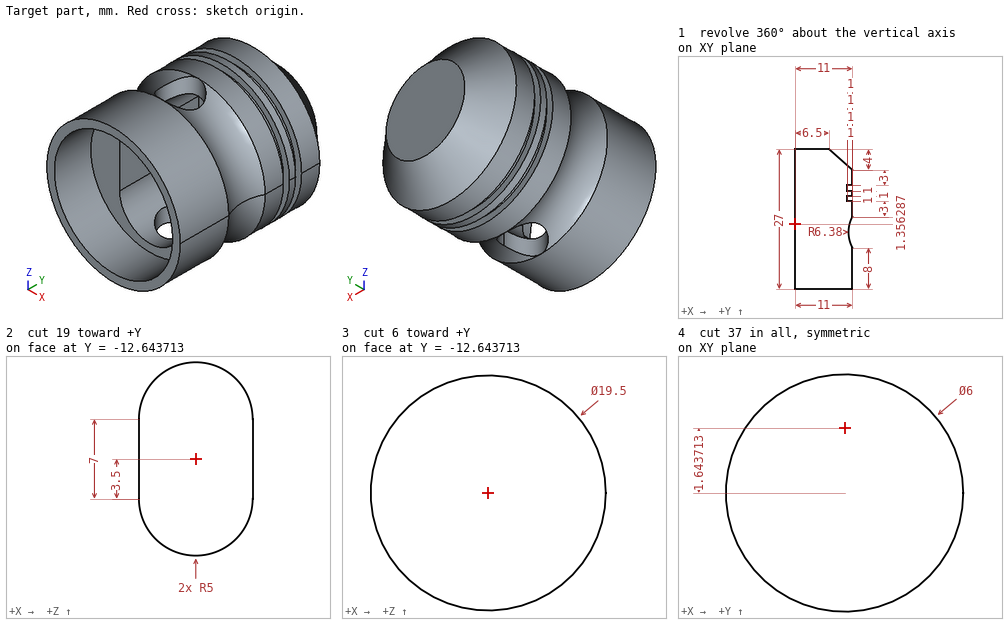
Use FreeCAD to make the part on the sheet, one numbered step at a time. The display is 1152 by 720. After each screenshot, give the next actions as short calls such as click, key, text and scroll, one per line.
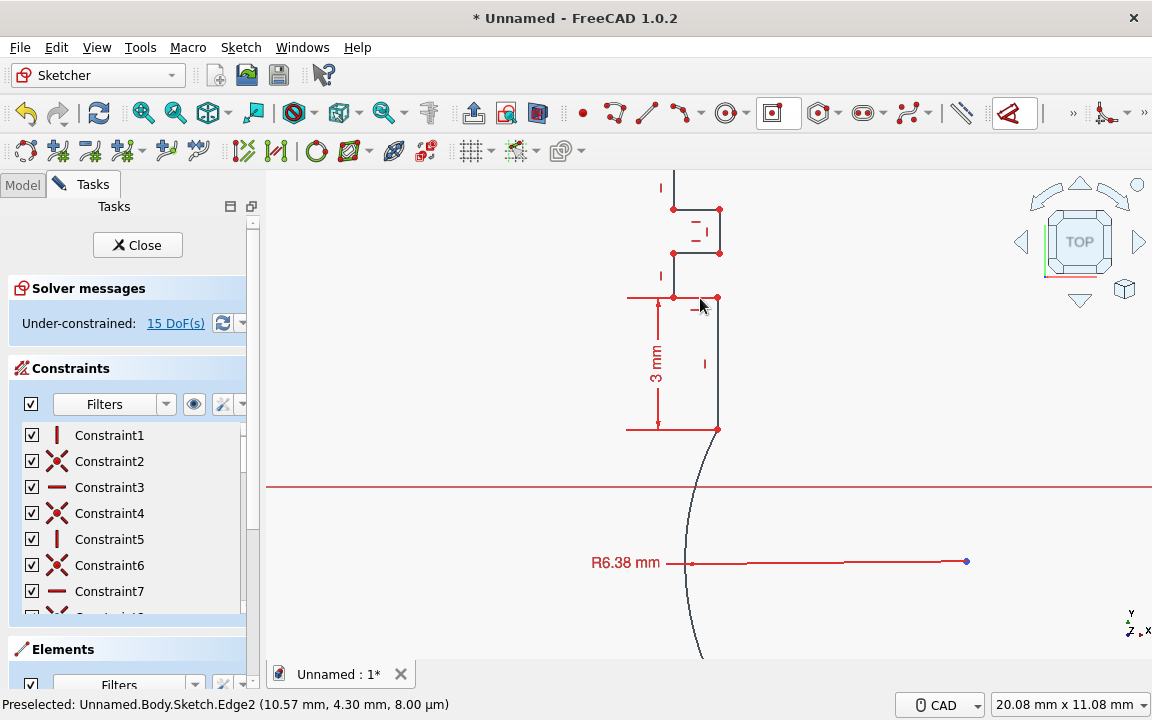
click(1032, 114)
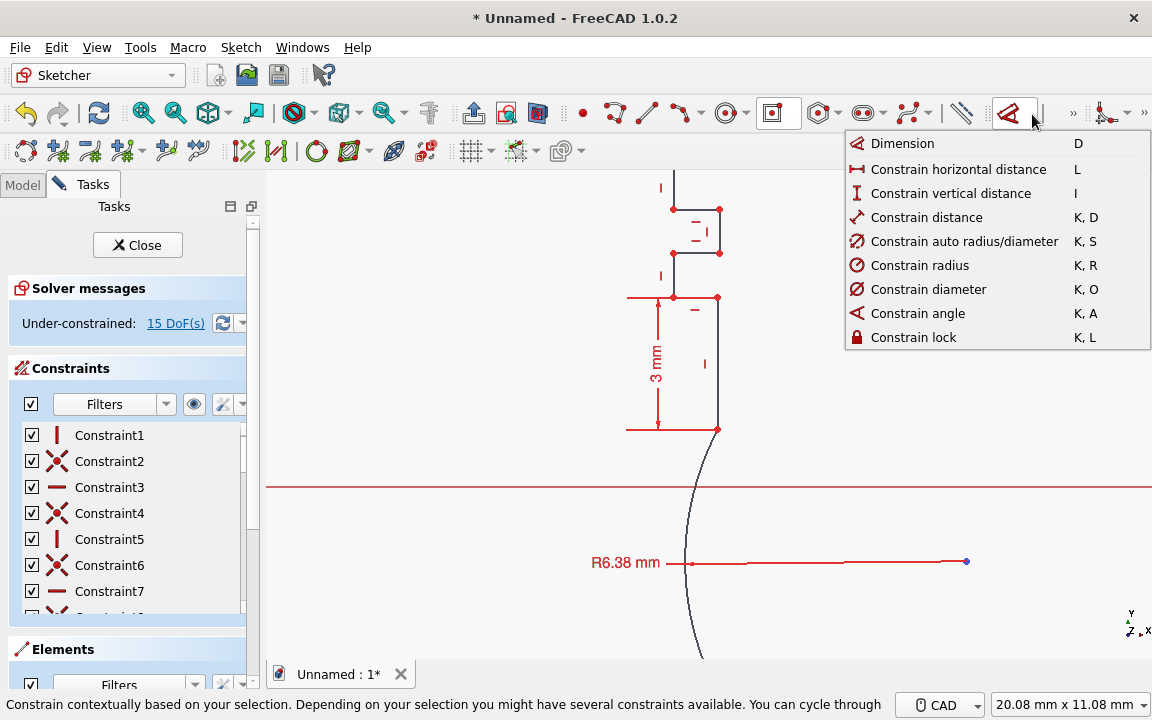
click(998, 169)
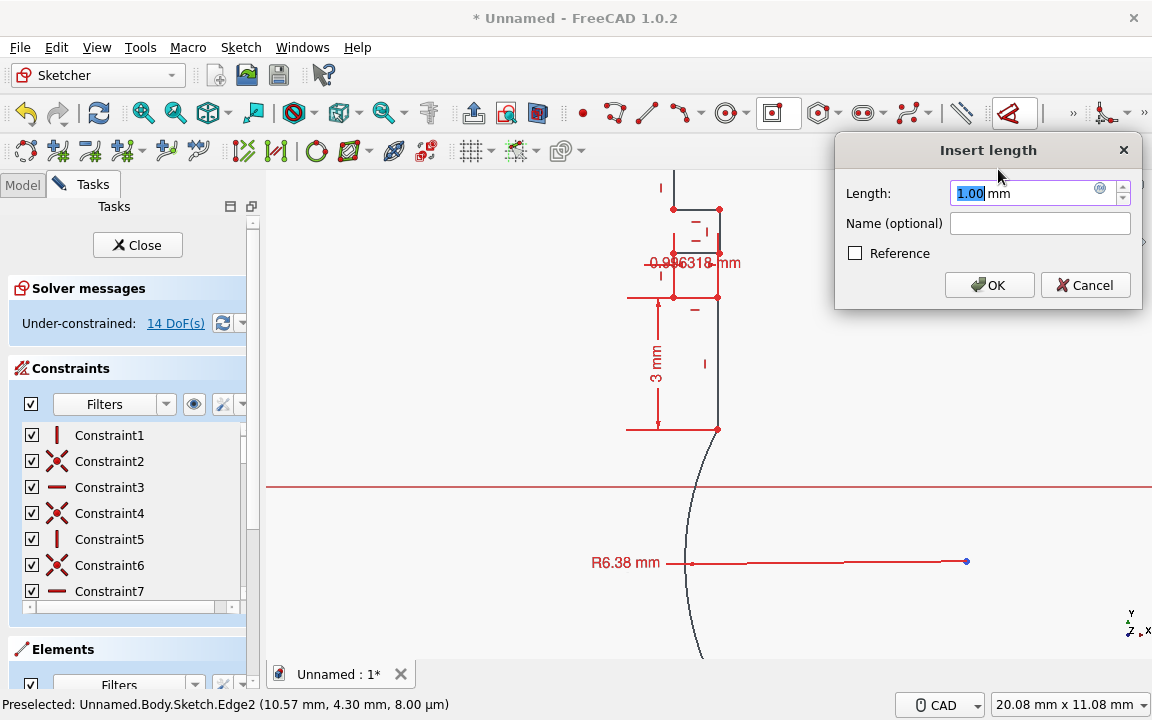
text(1)
key(Return)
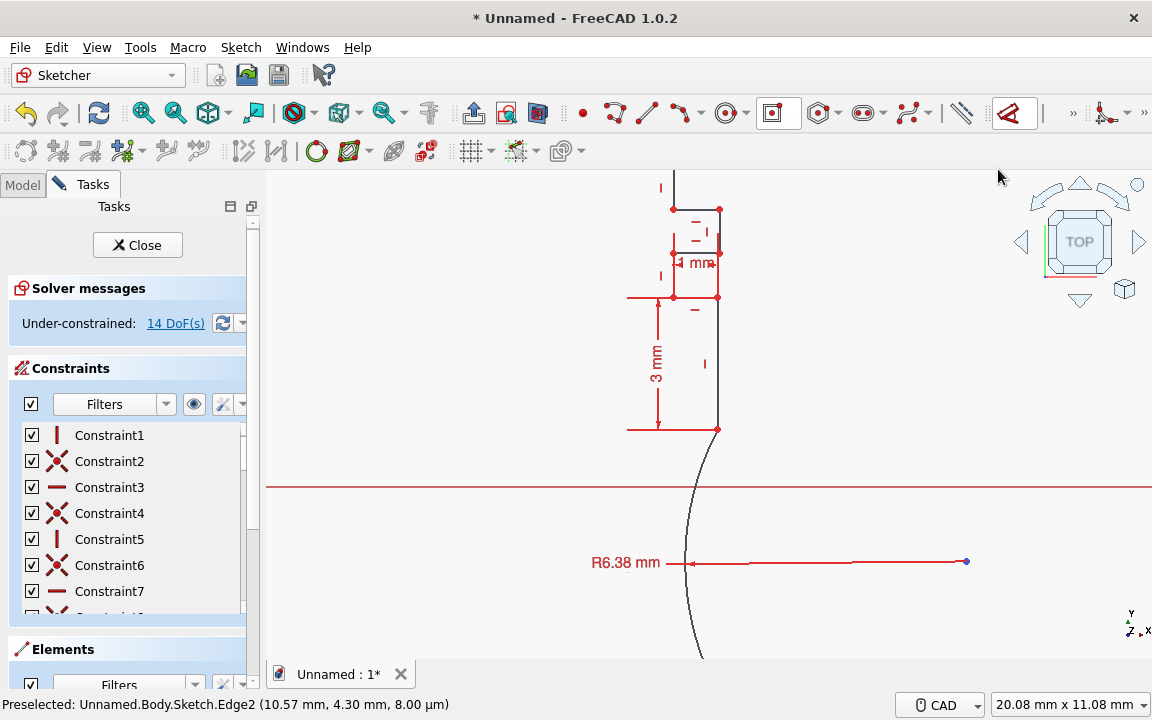
click(674, 284)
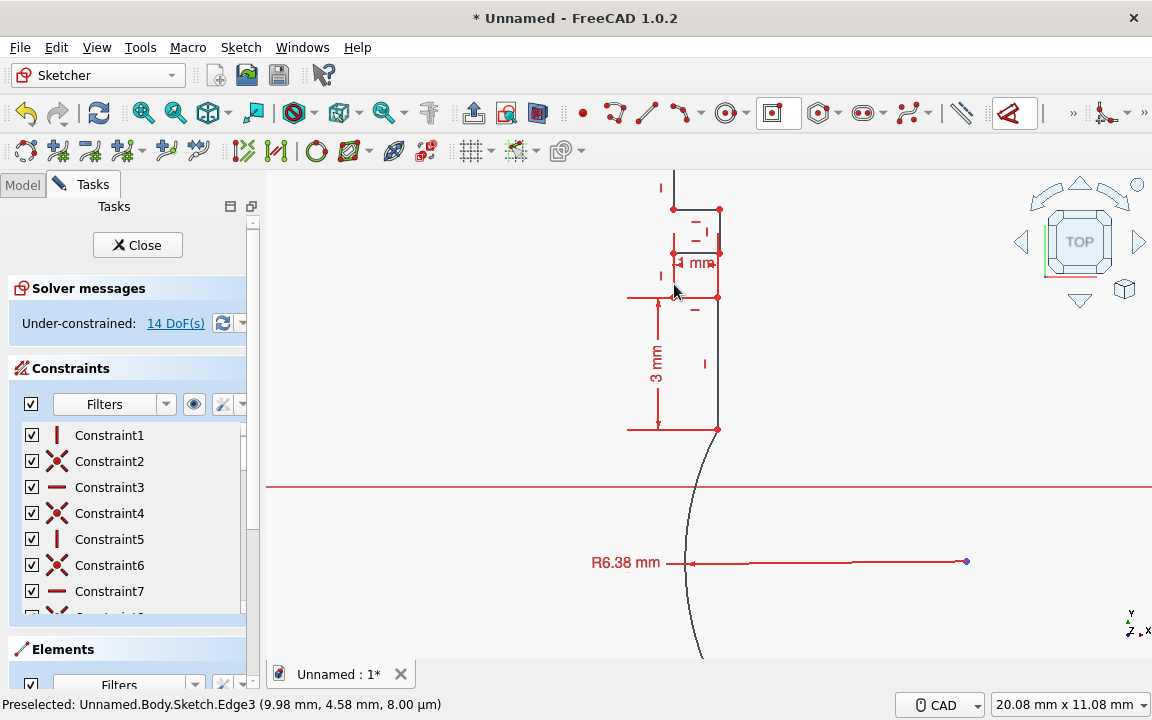
key(i)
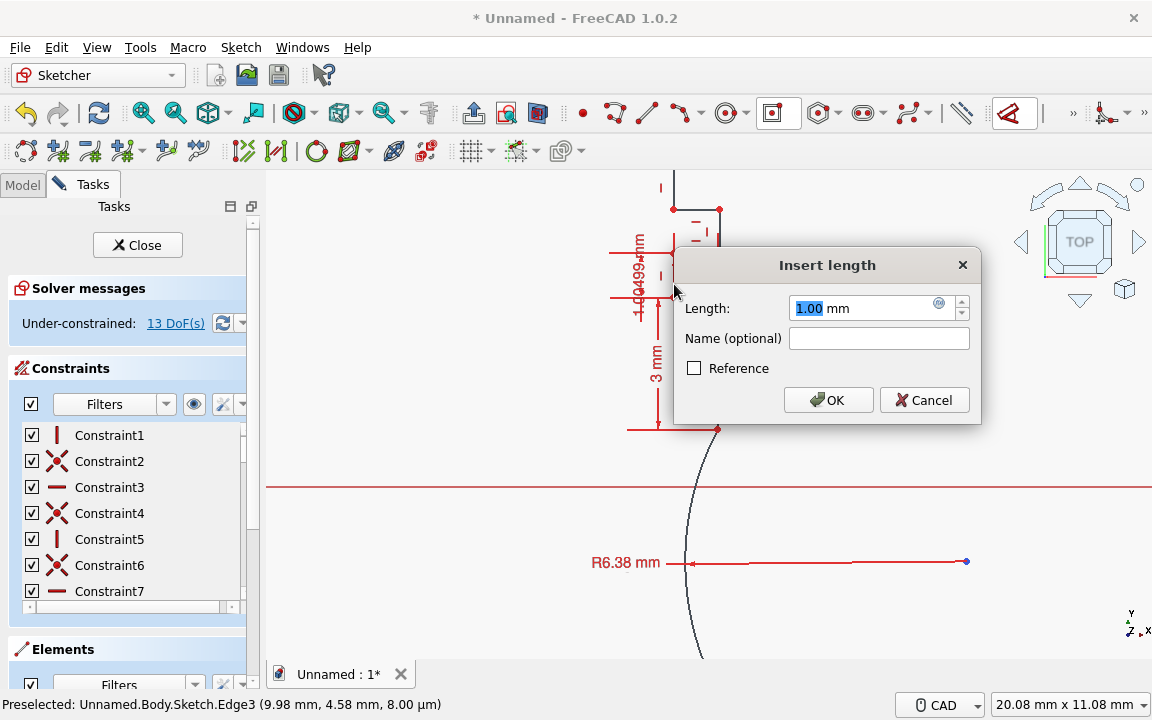
text(1)
key(Return)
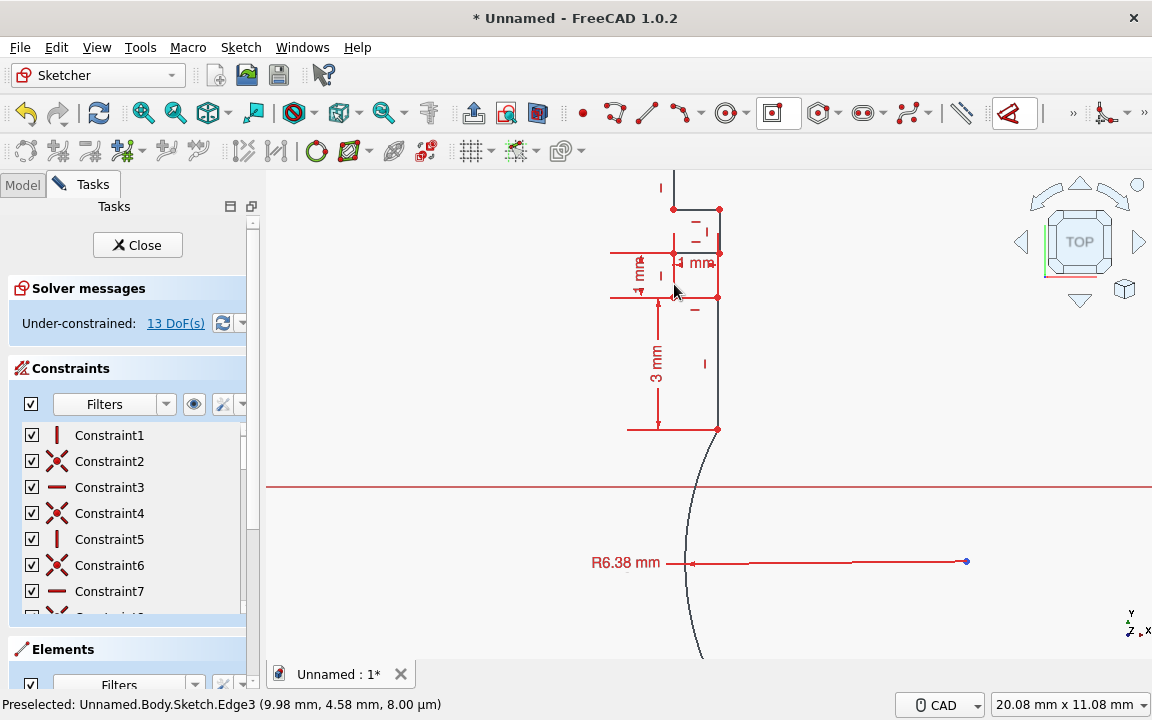
click(688, 253)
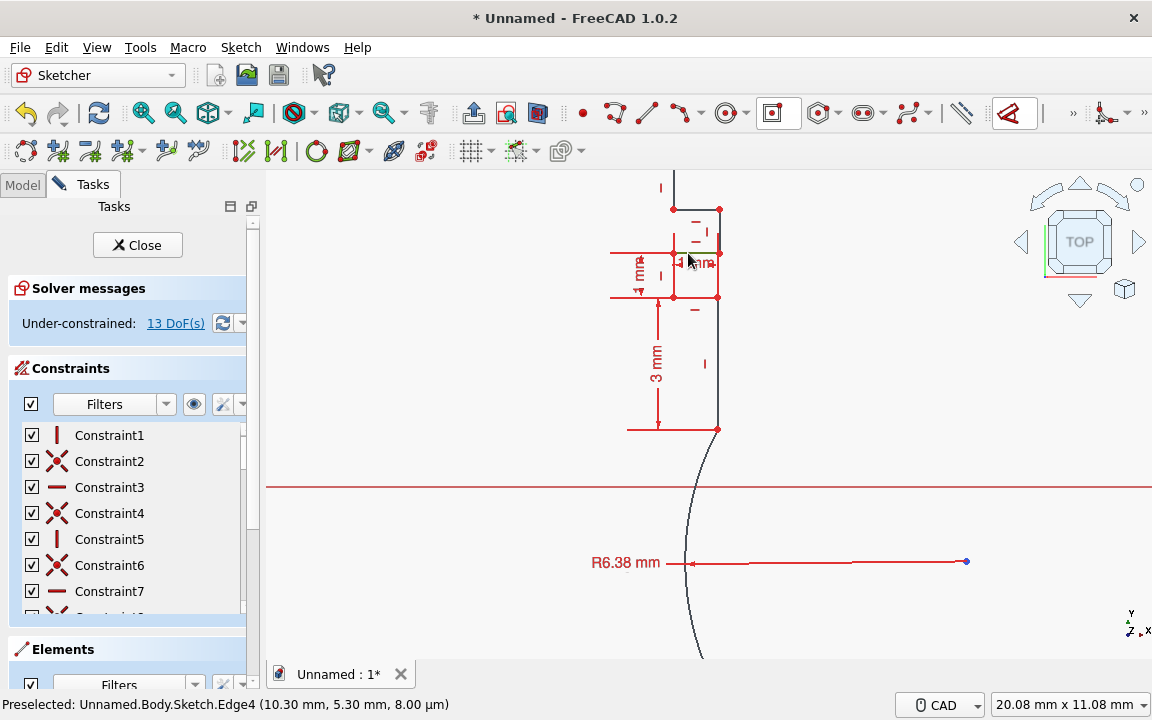
key(l)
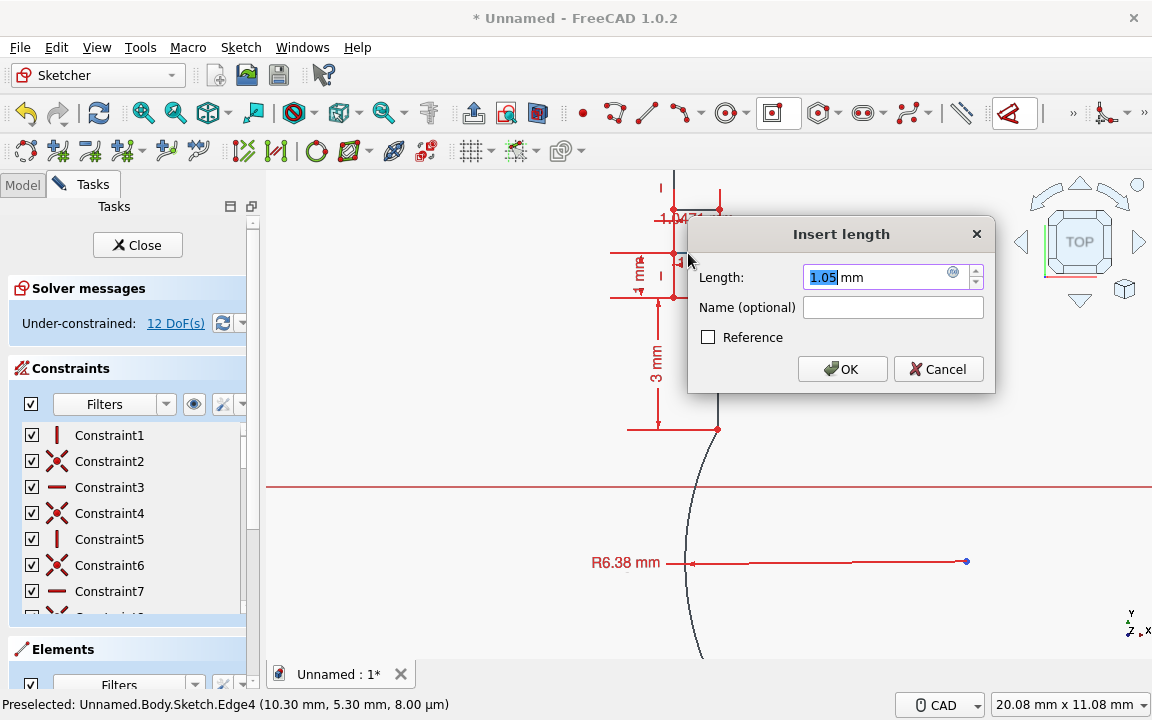
text(1)
key(Return)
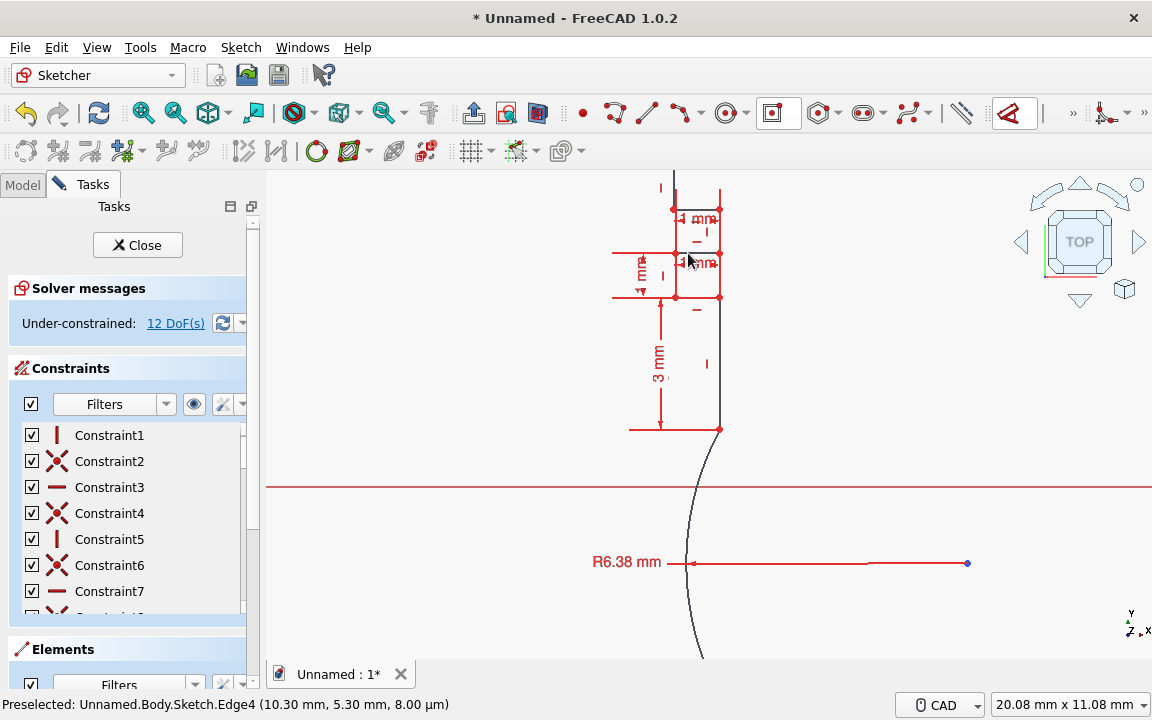
click(720, 240)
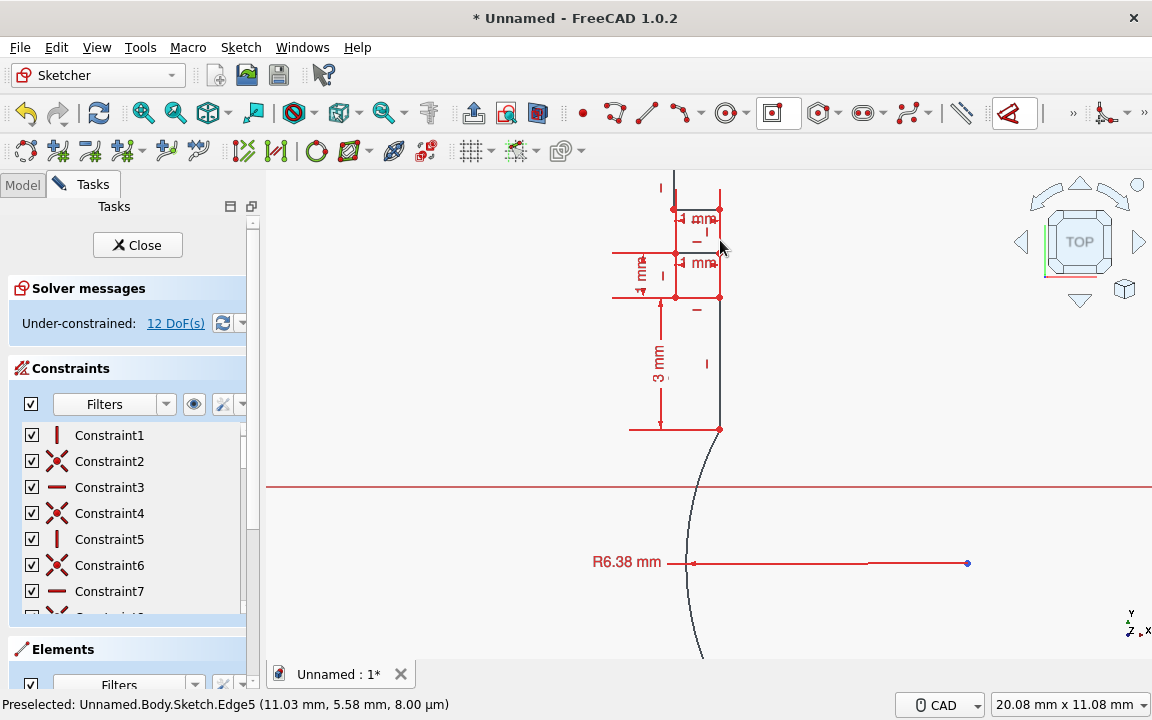
key(i)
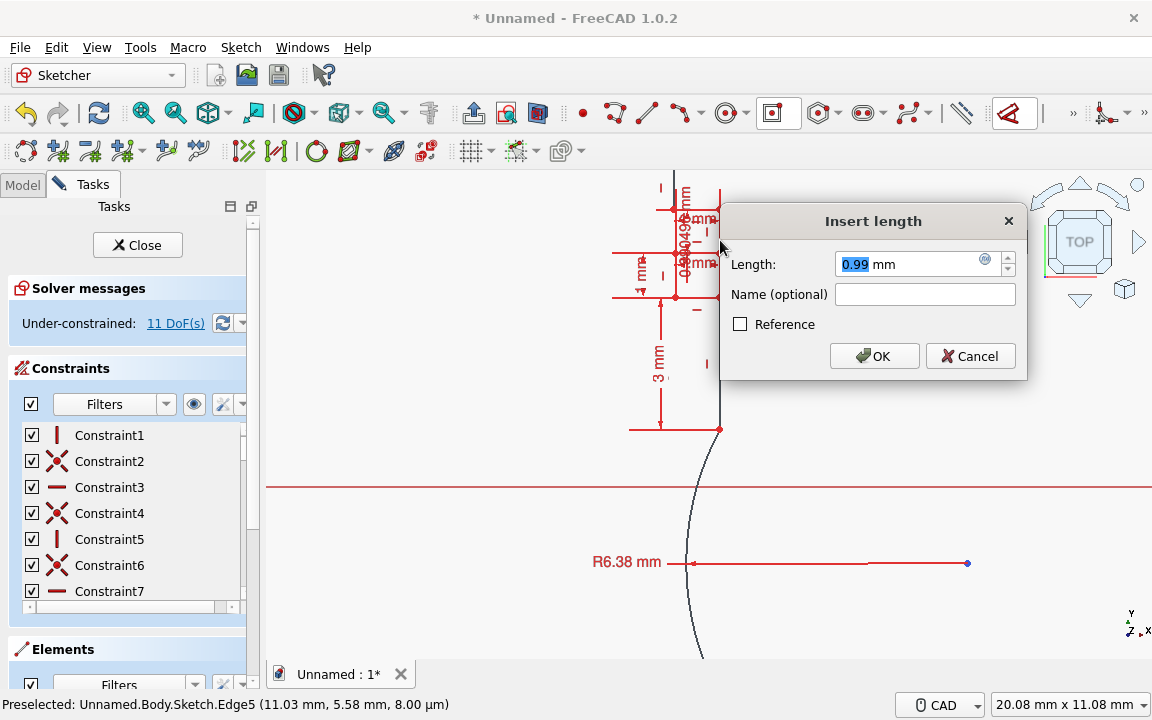
text(1)
key(Return)